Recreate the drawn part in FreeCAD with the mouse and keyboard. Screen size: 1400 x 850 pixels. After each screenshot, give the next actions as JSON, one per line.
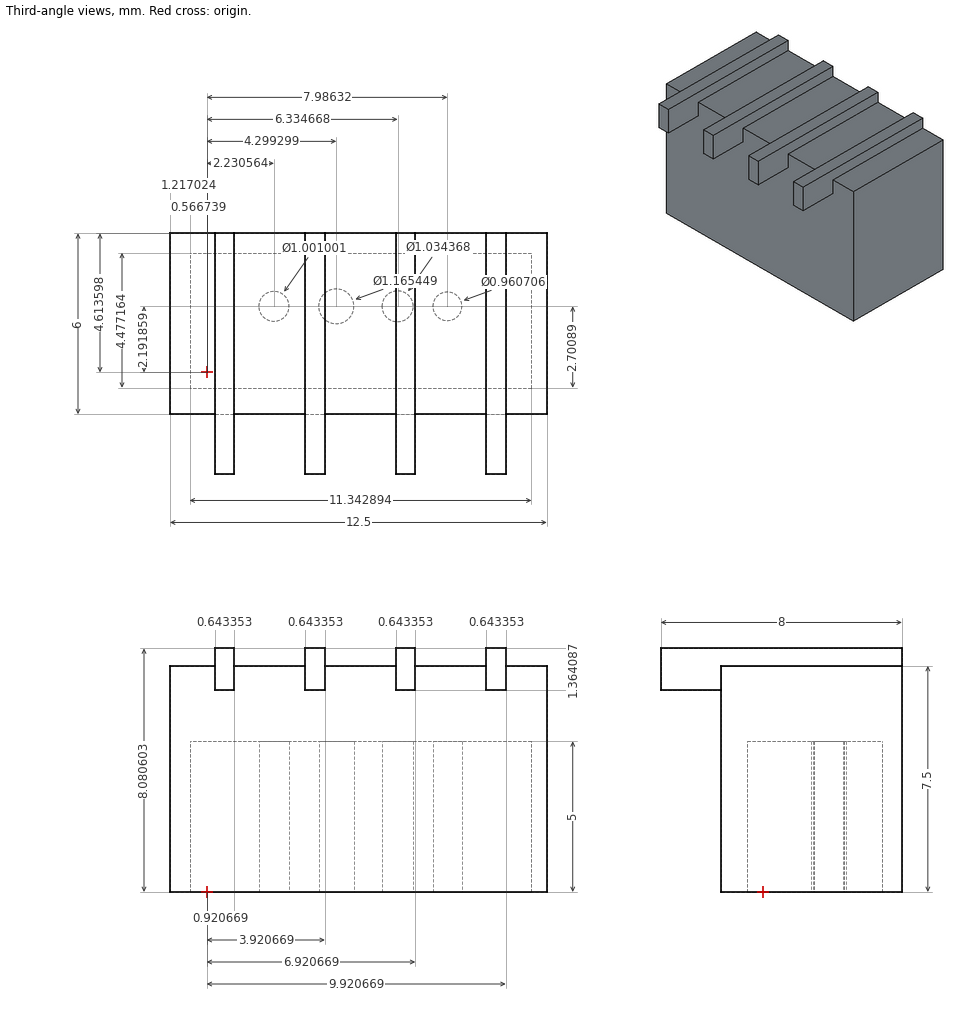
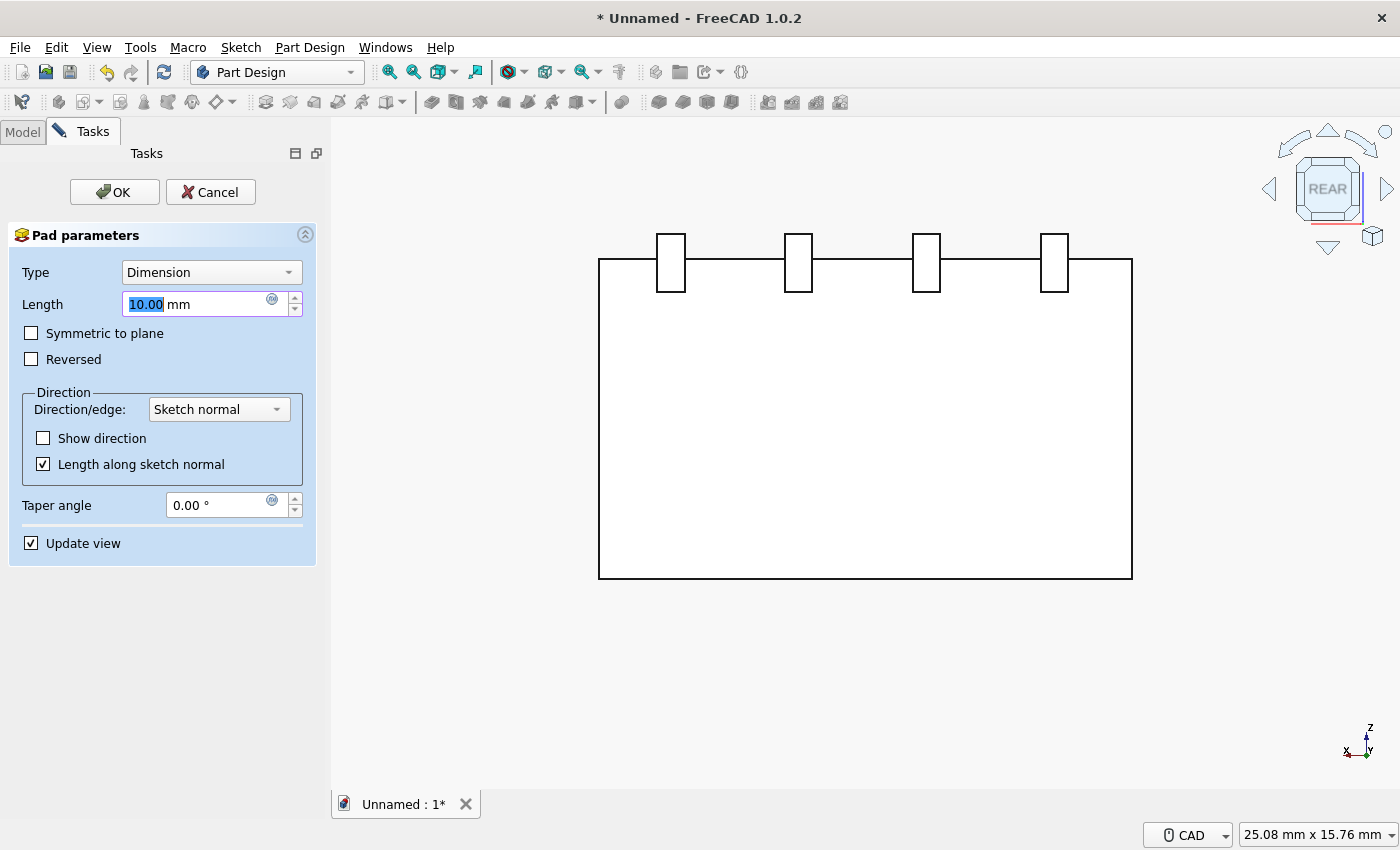
{"action": "type", "text": "8"}
{"action": "key", "text": "Tab"}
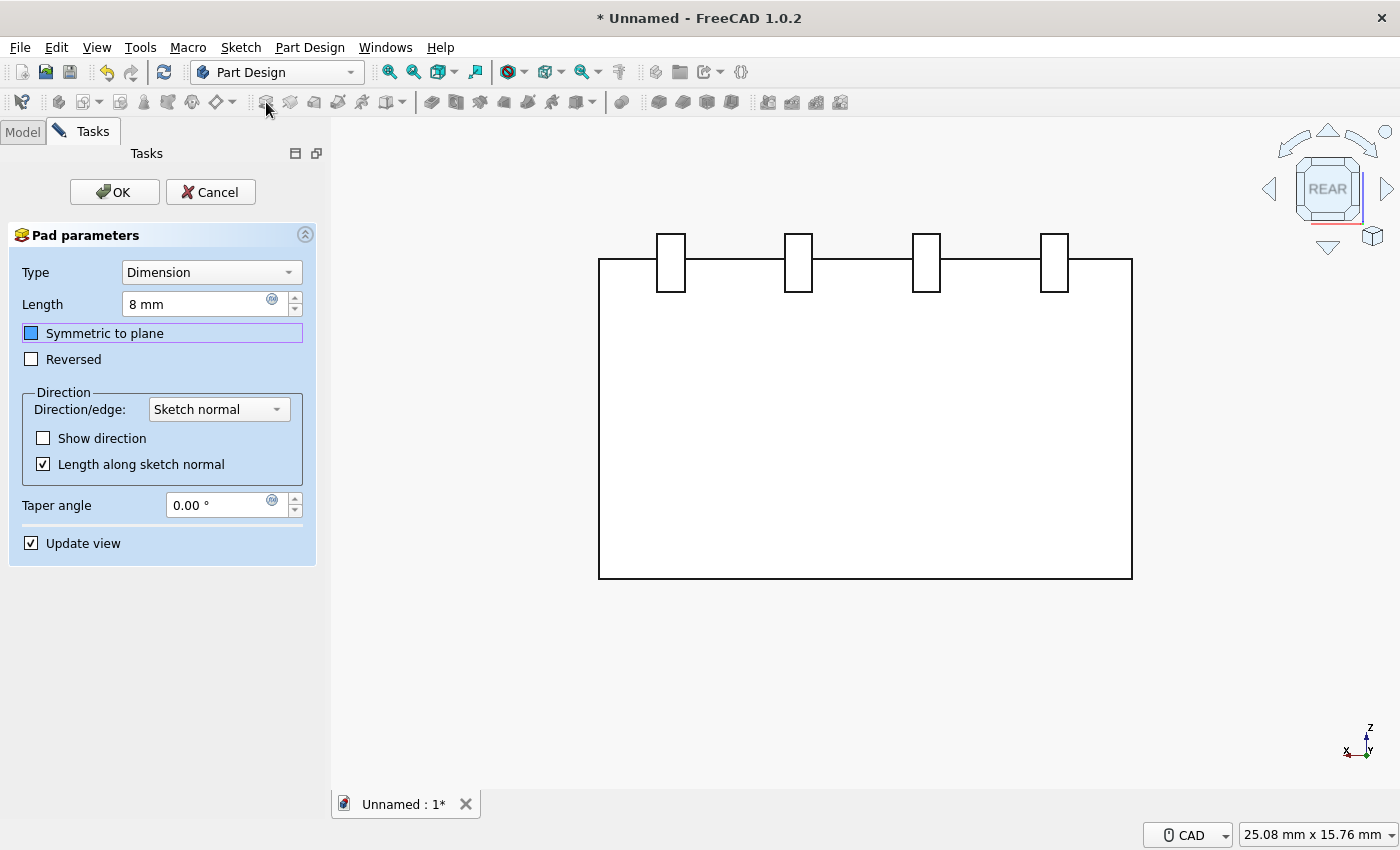
{"action": "left_click", "coordinate": [30, 359]}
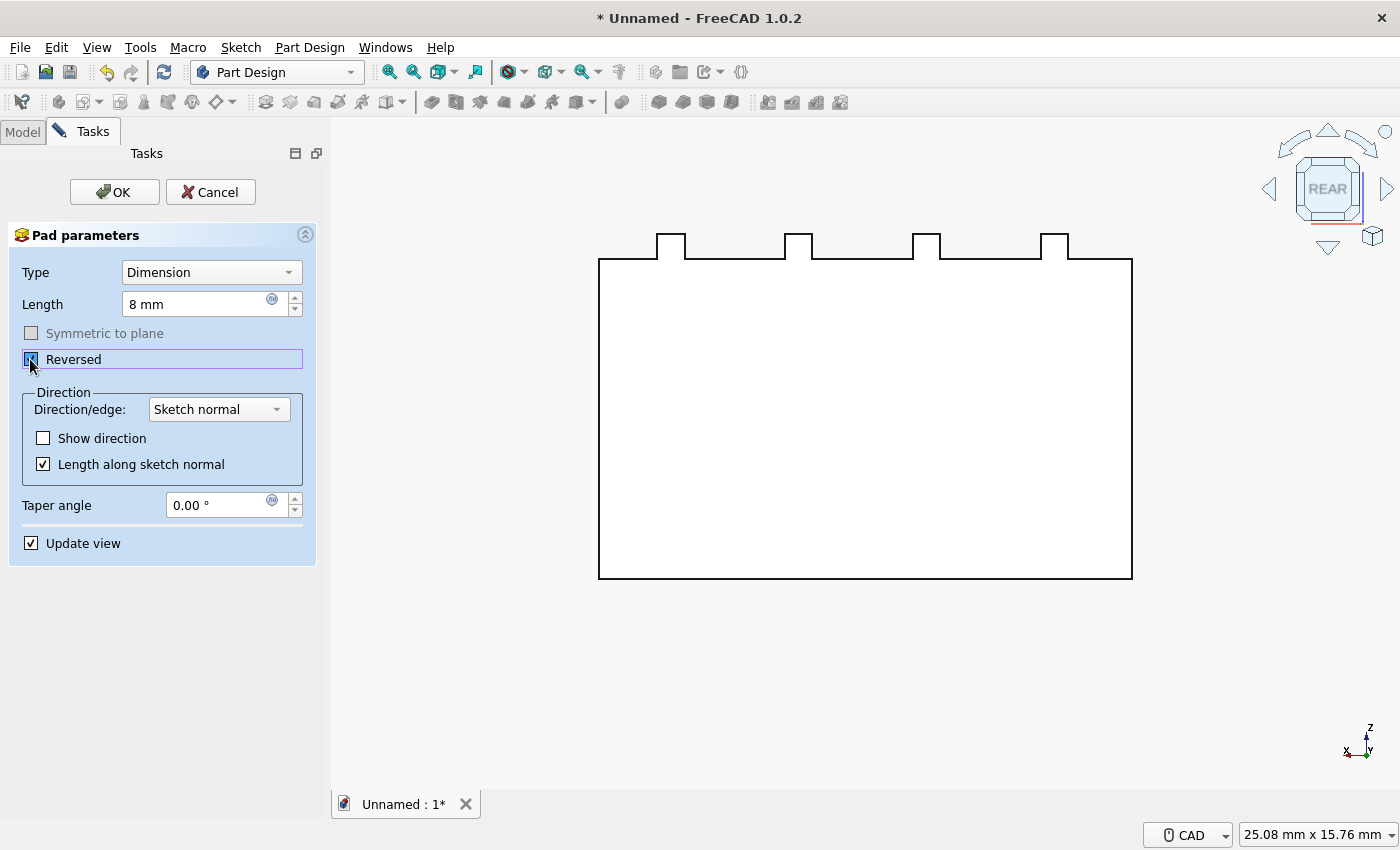
{"action": "left_click", "coordinate": [115, 192]}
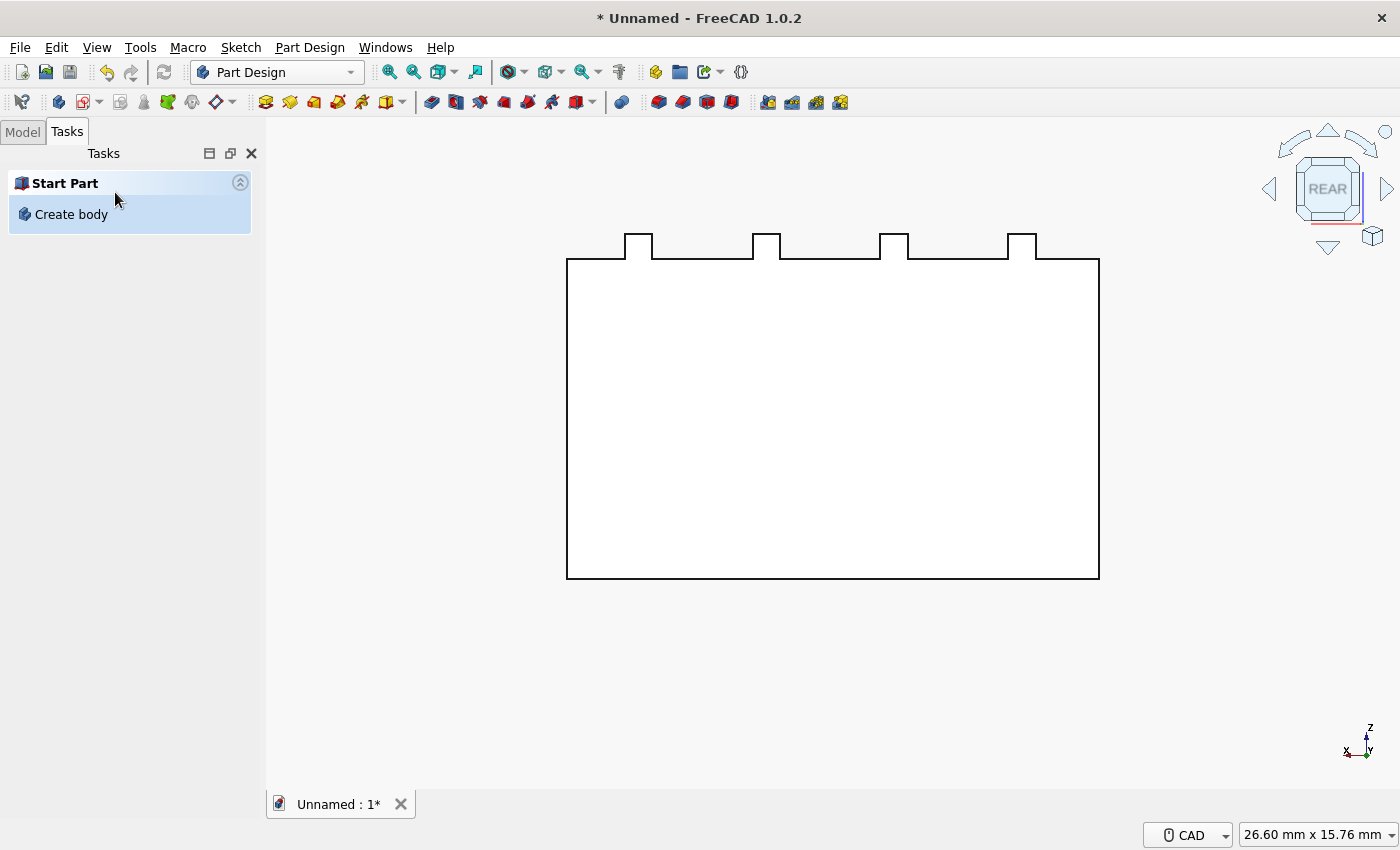
{"action": "key", "text": "0"}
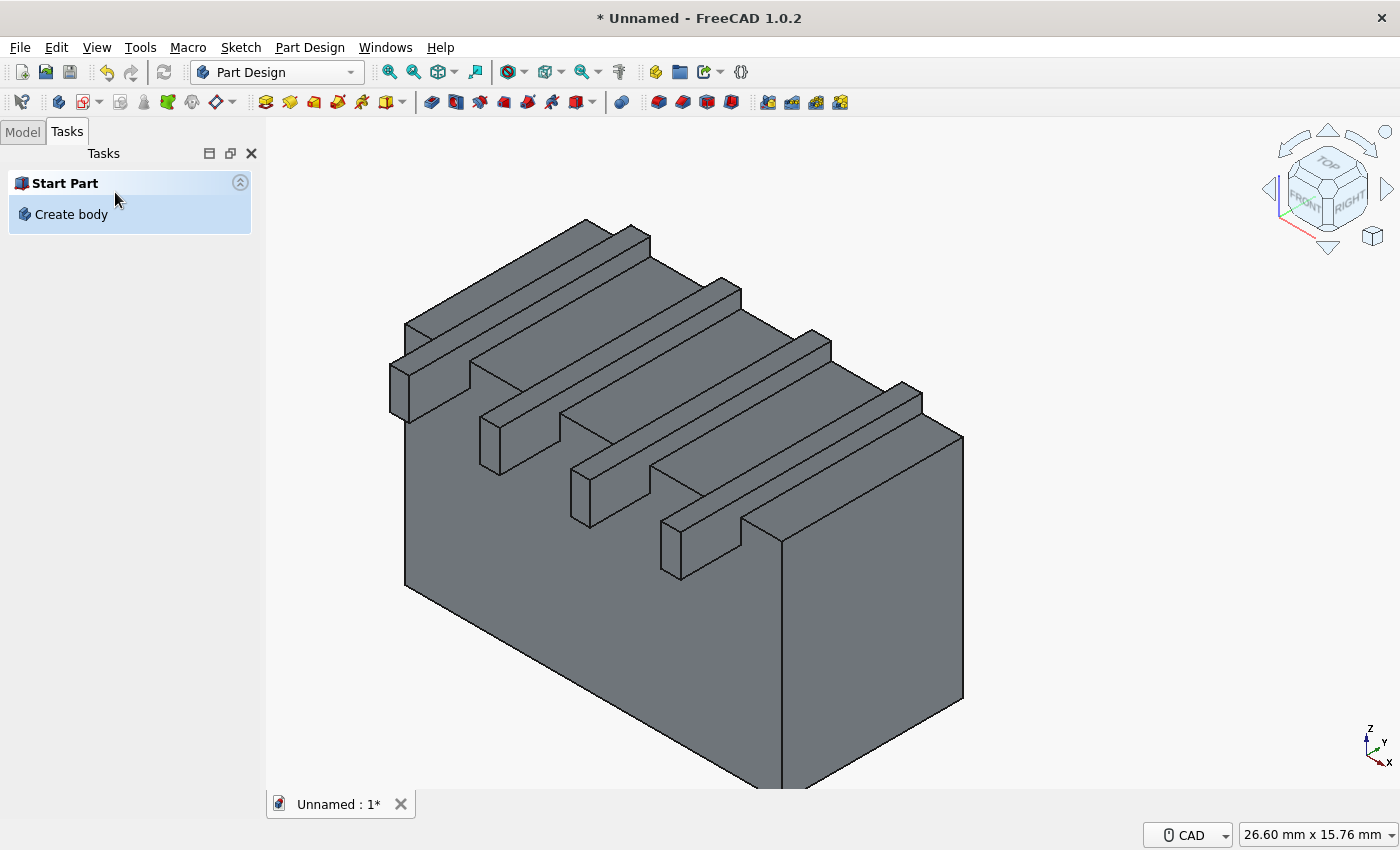
{"action": "left_click", "coordinate": [390, 72]}